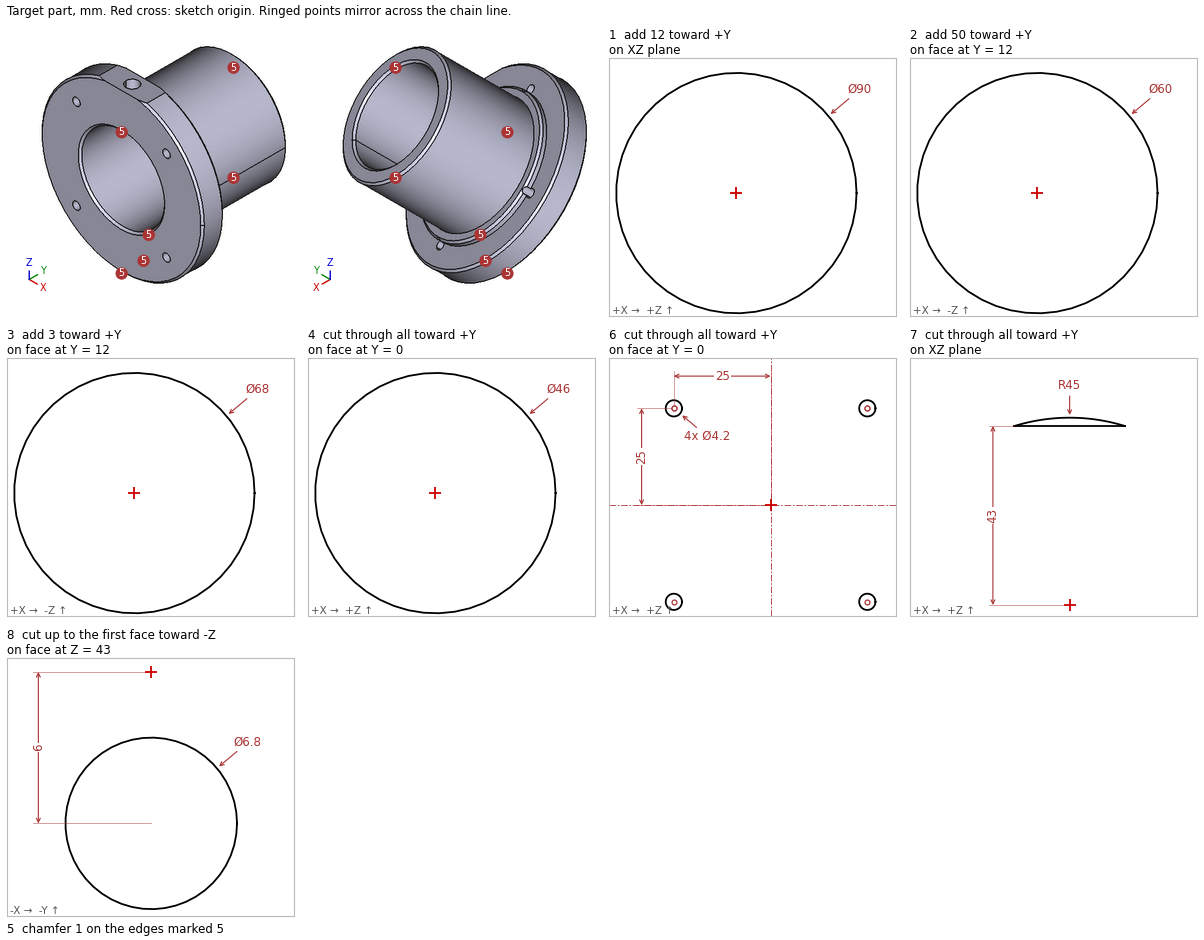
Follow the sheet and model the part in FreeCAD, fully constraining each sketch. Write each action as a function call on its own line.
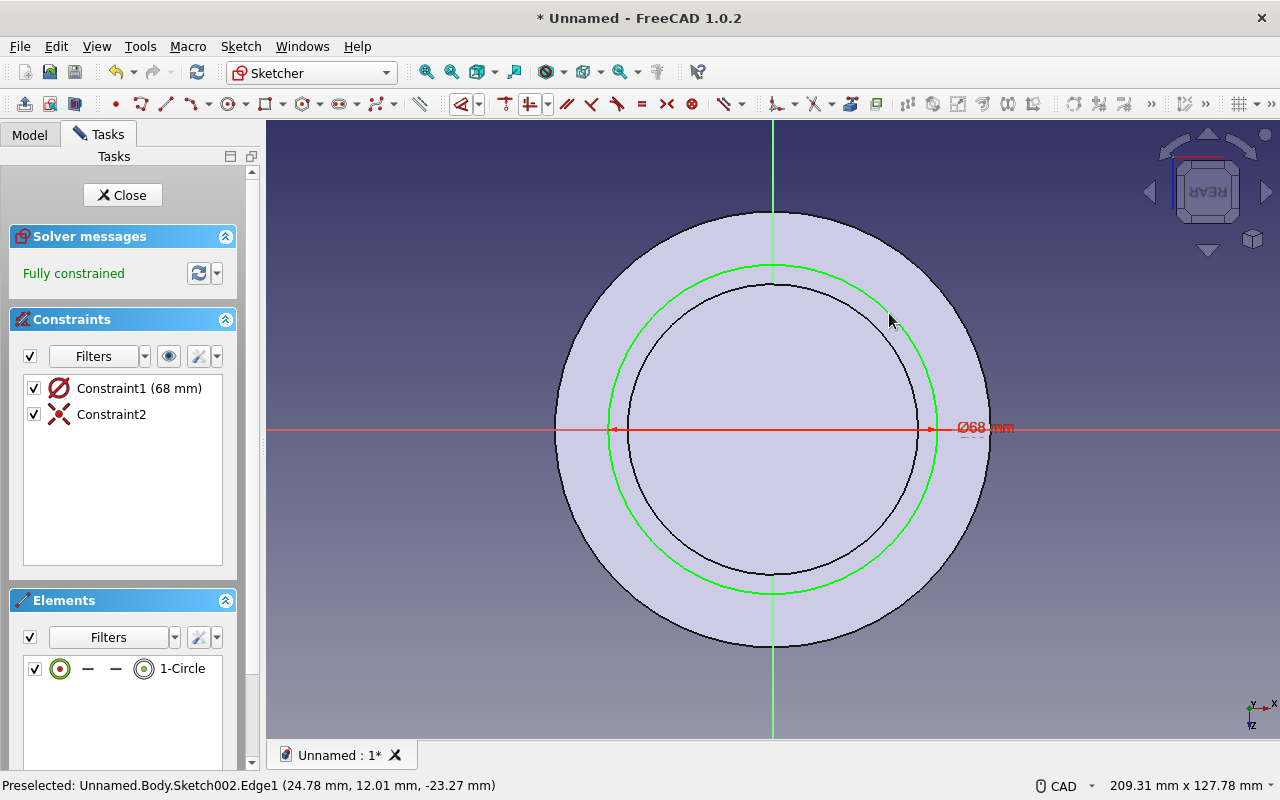
click(123, 195)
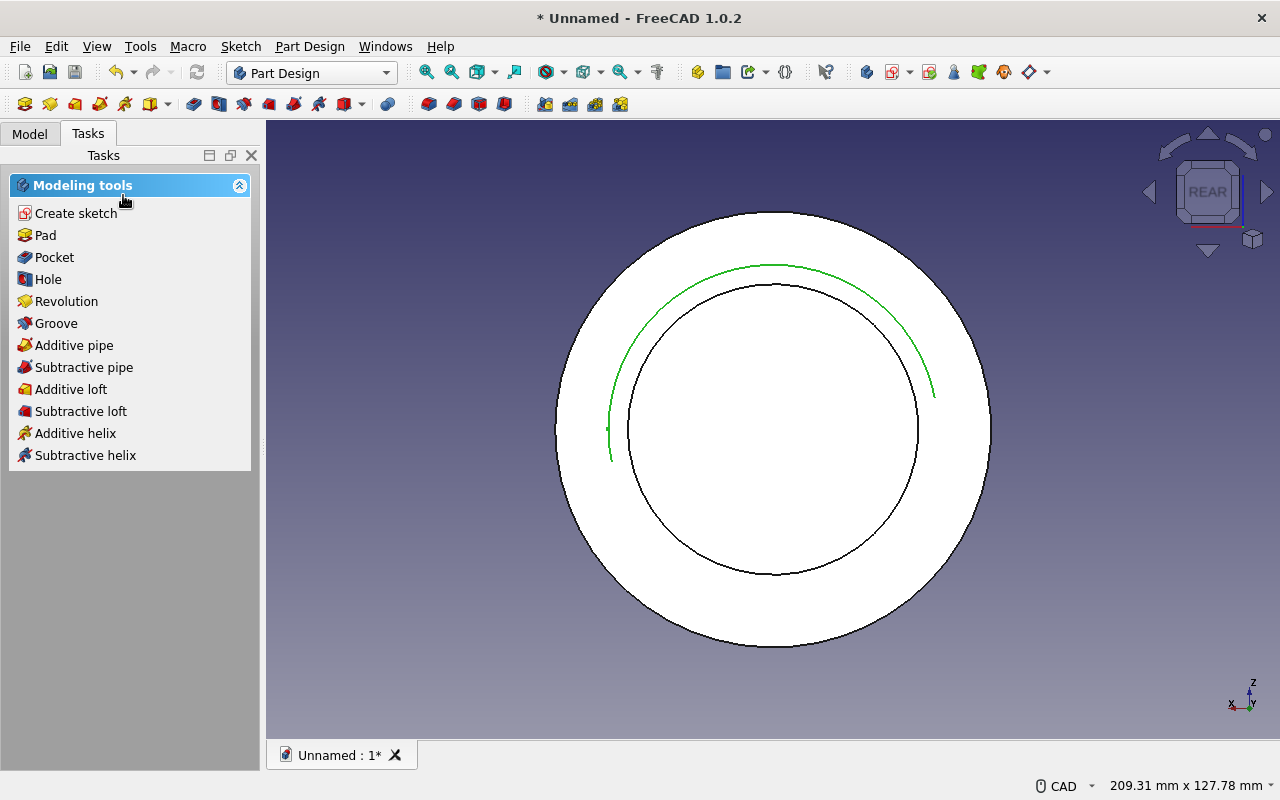
click(25, 104)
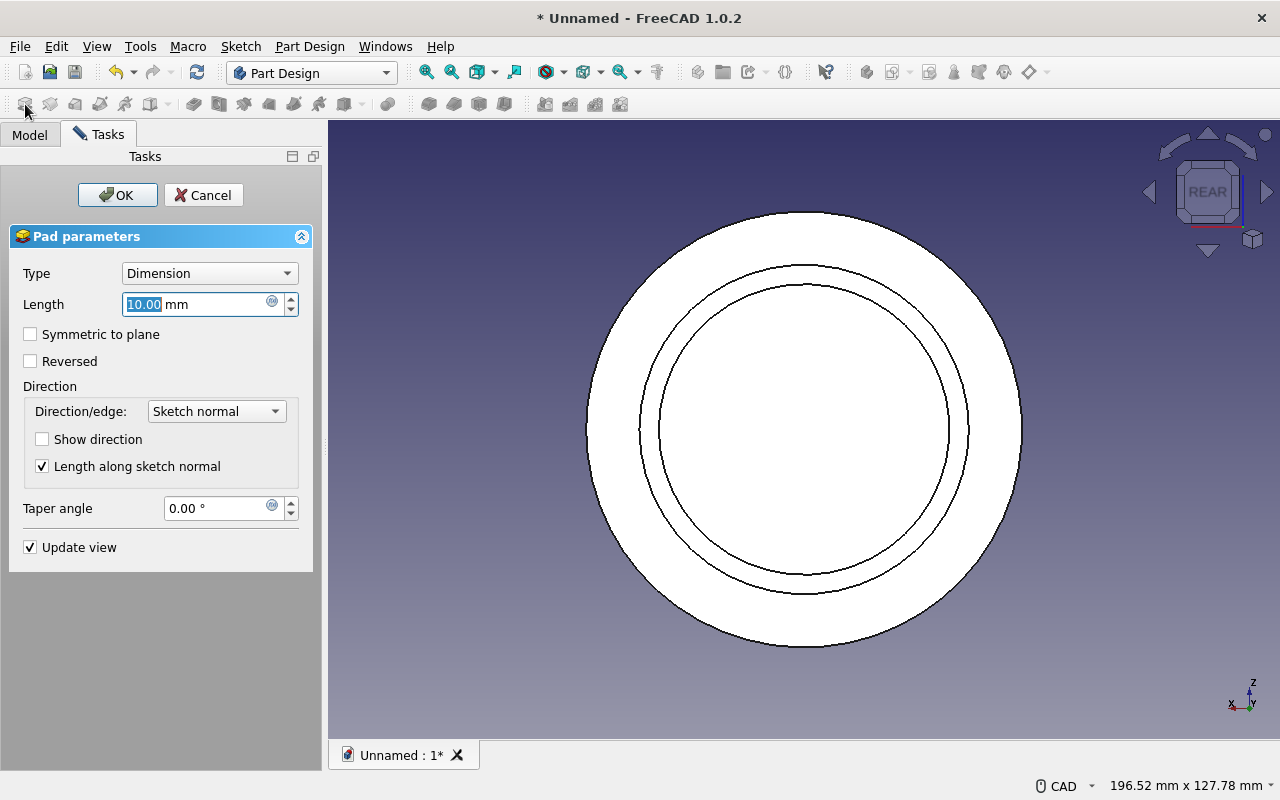
text(3)
key(Tab)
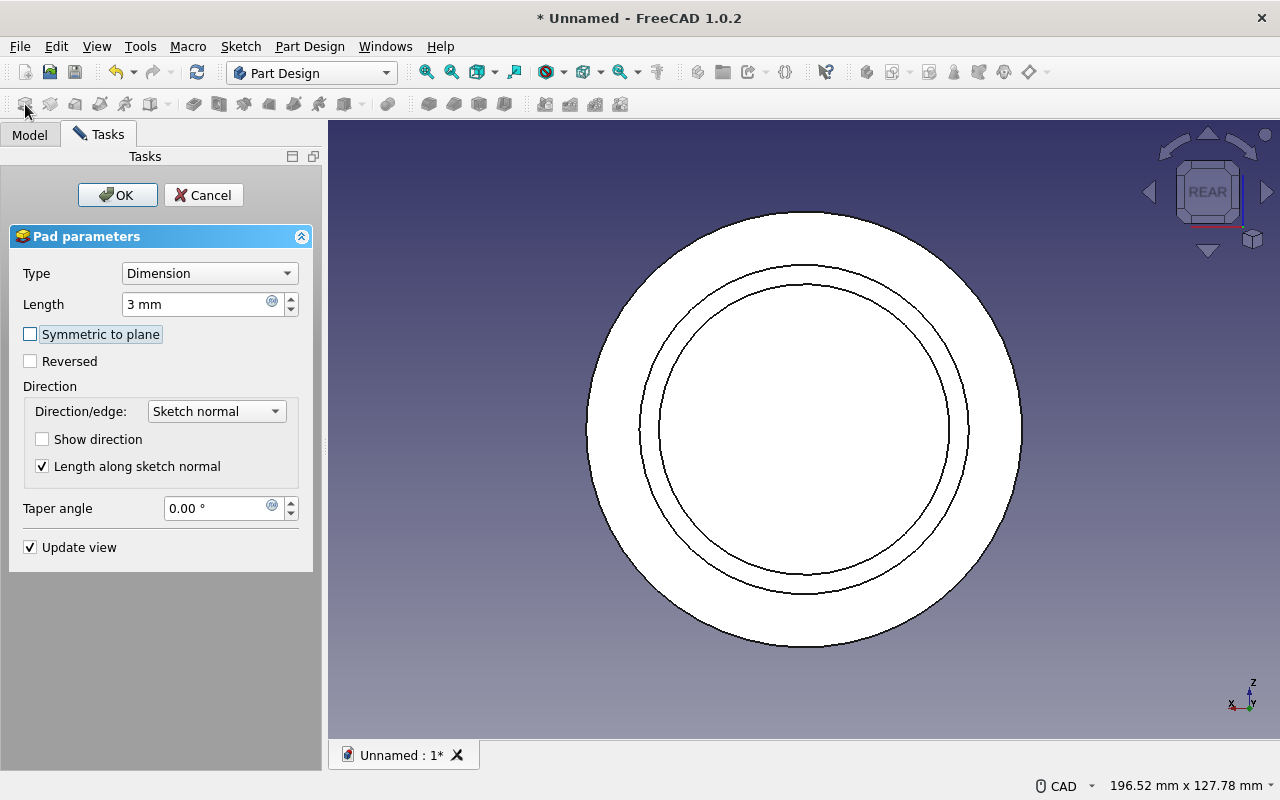
click(118, 195)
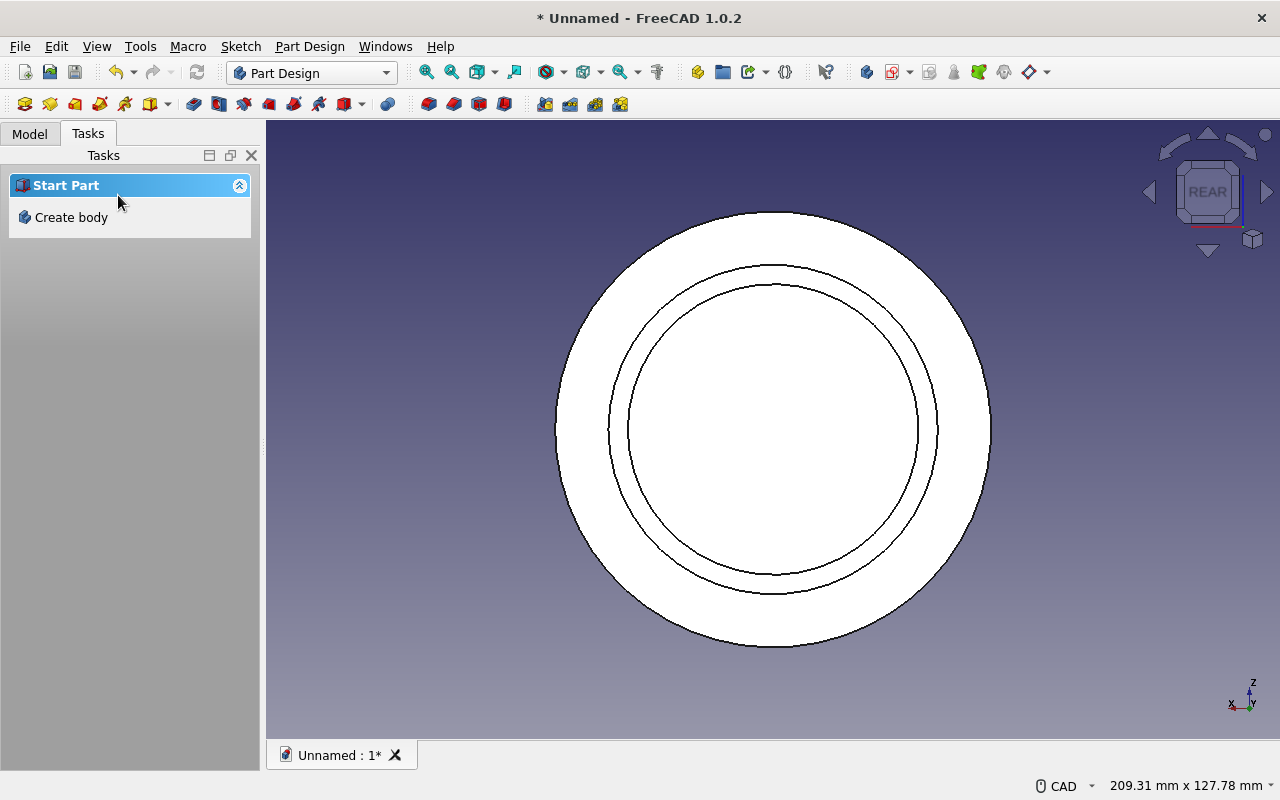
key(0)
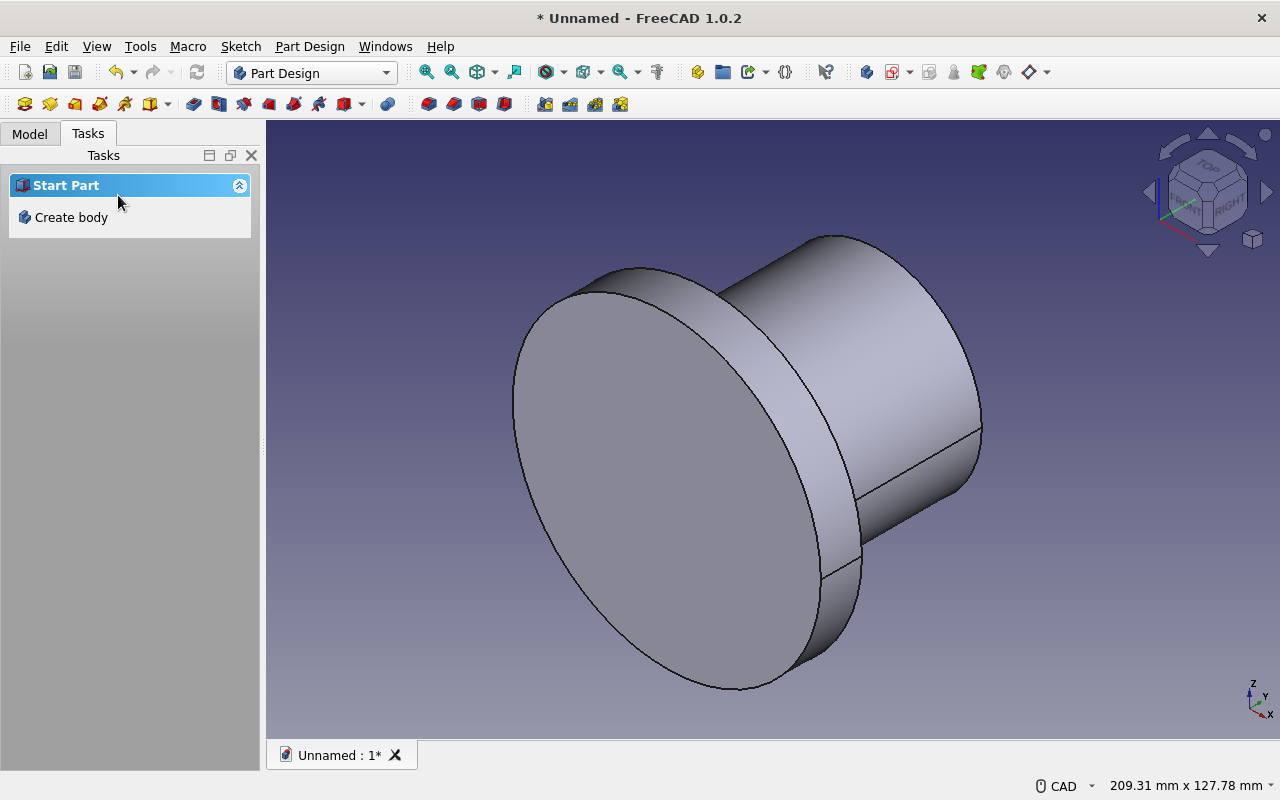
click(427, 72)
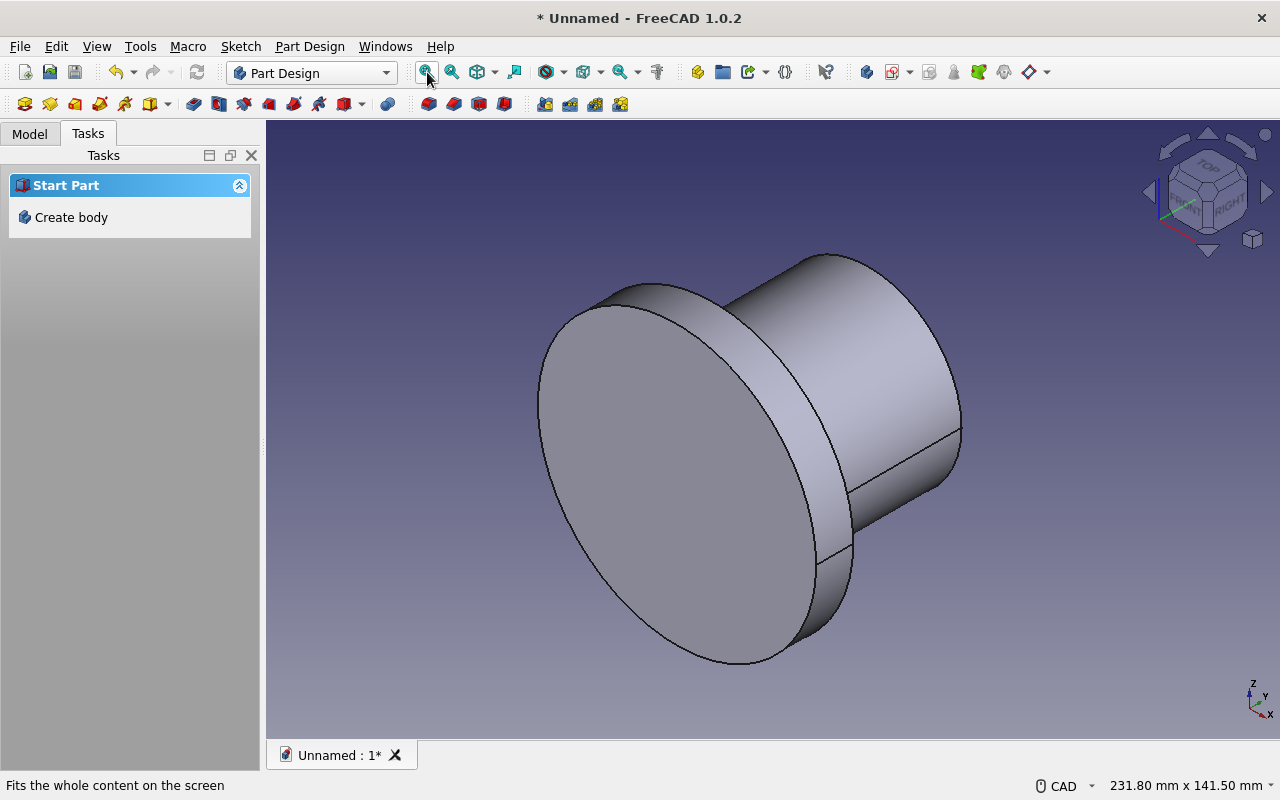
click(677, 484)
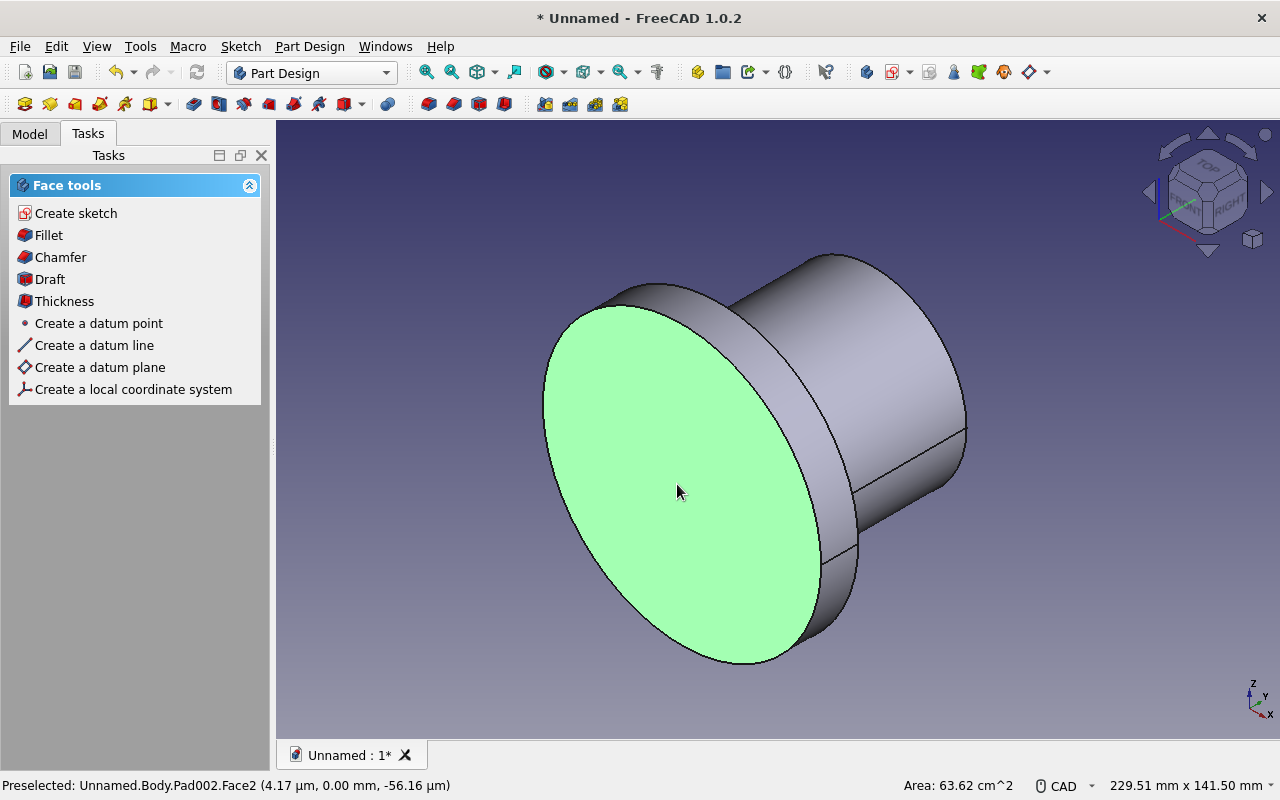
click(892, 72)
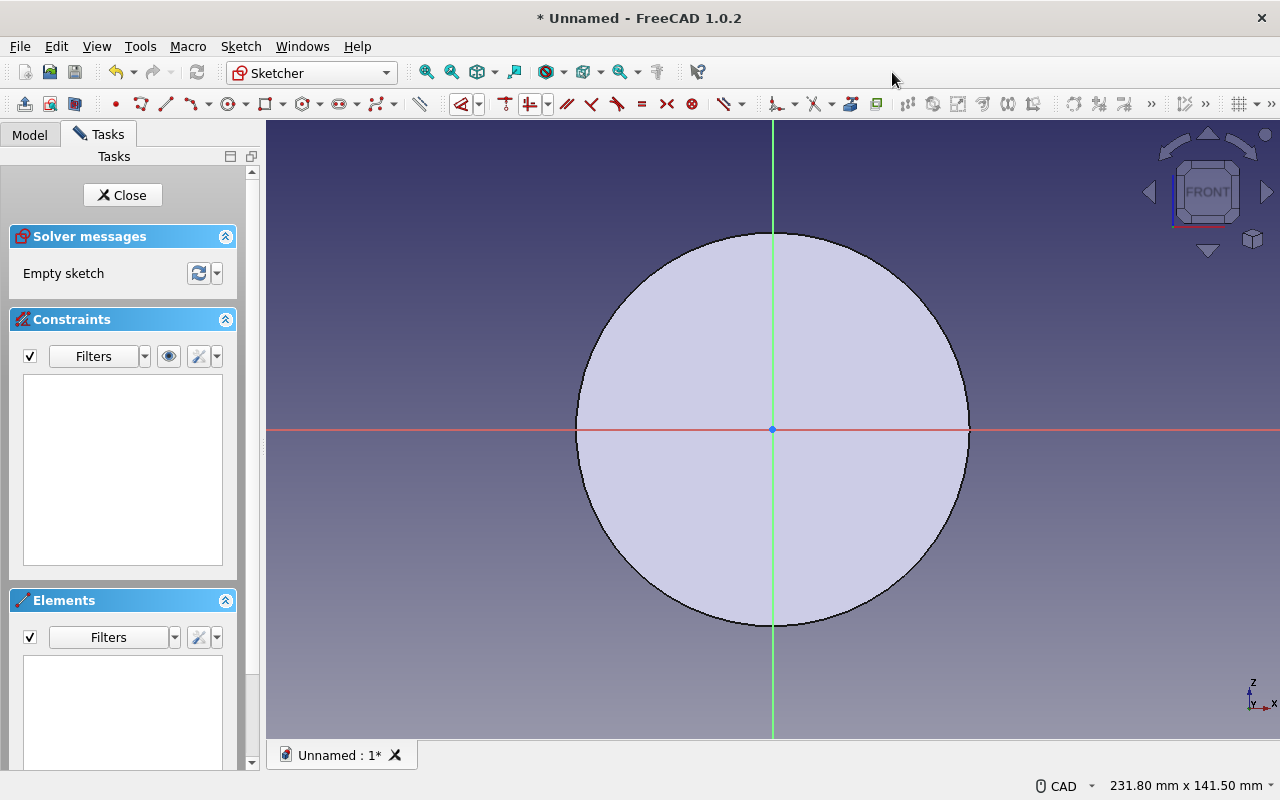
scroll(856, 430, up, 3)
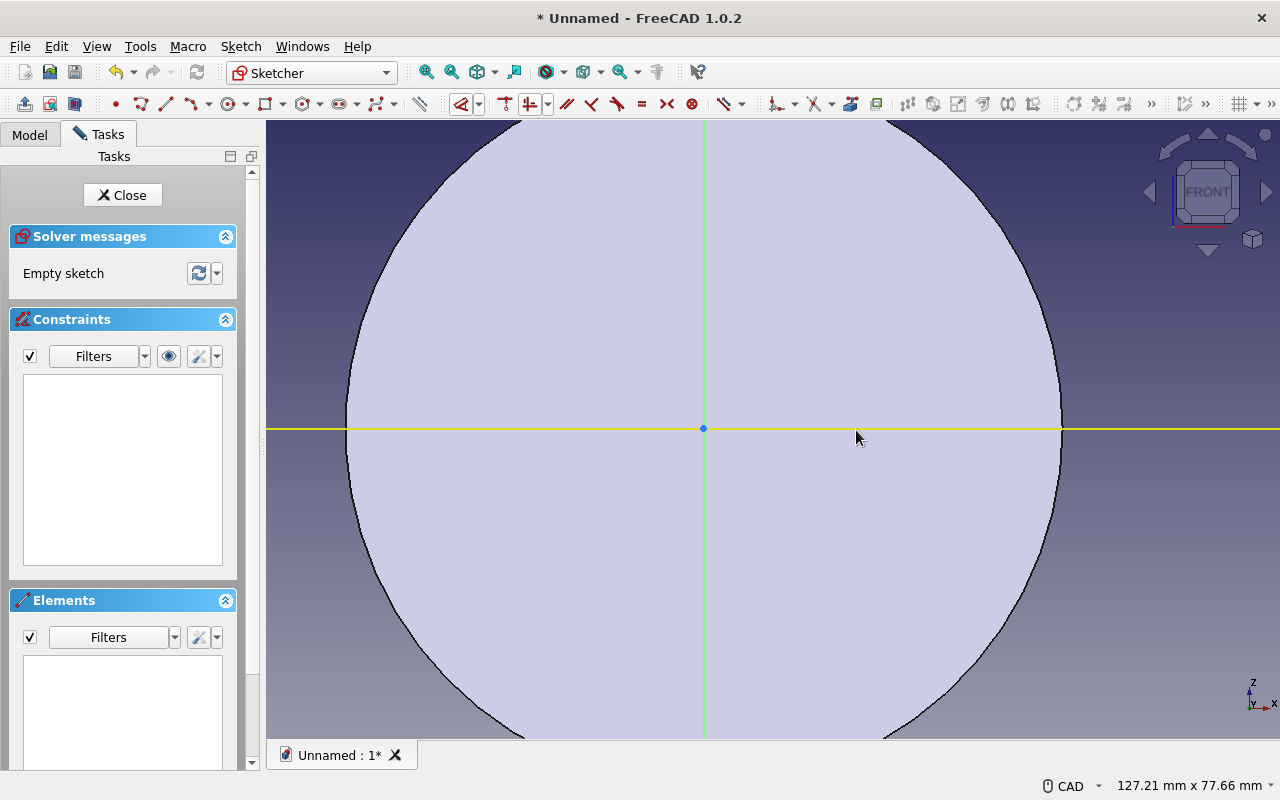
click(228, 104)